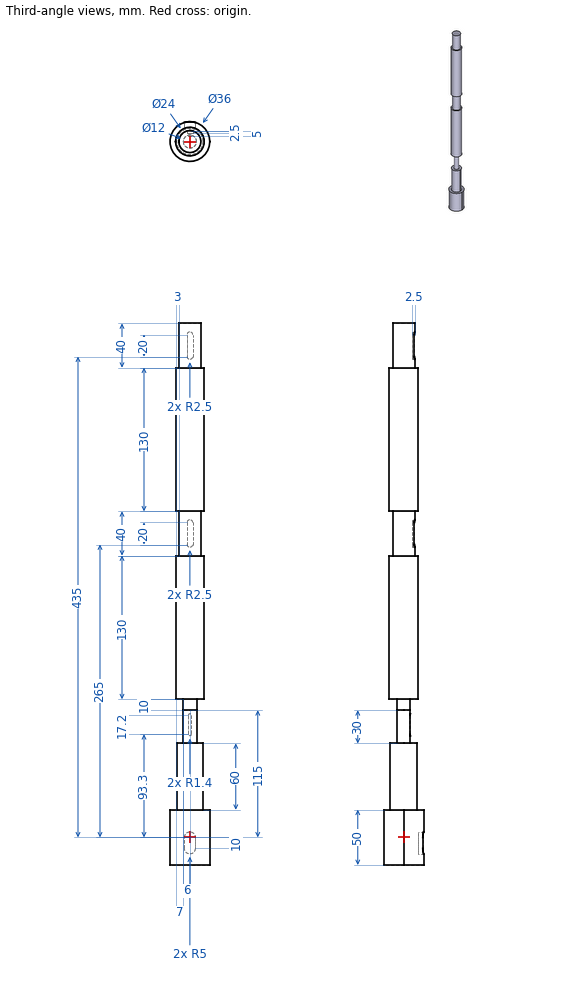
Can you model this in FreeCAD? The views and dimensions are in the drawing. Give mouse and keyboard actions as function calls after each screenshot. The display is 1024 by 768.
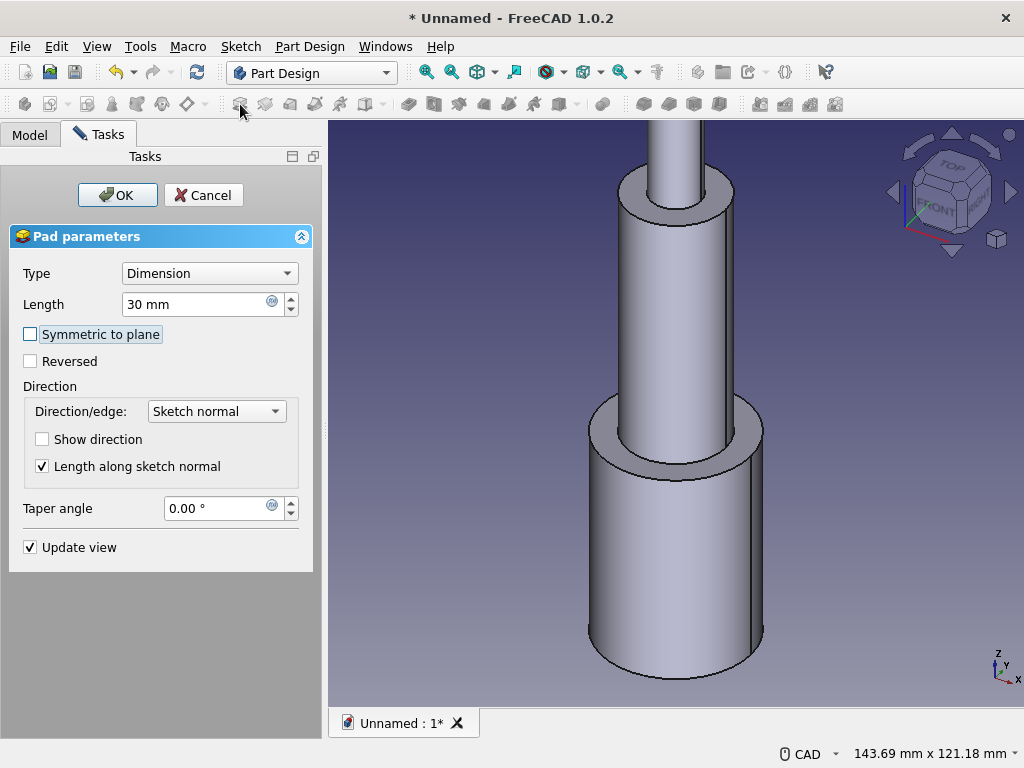
click(118, 195)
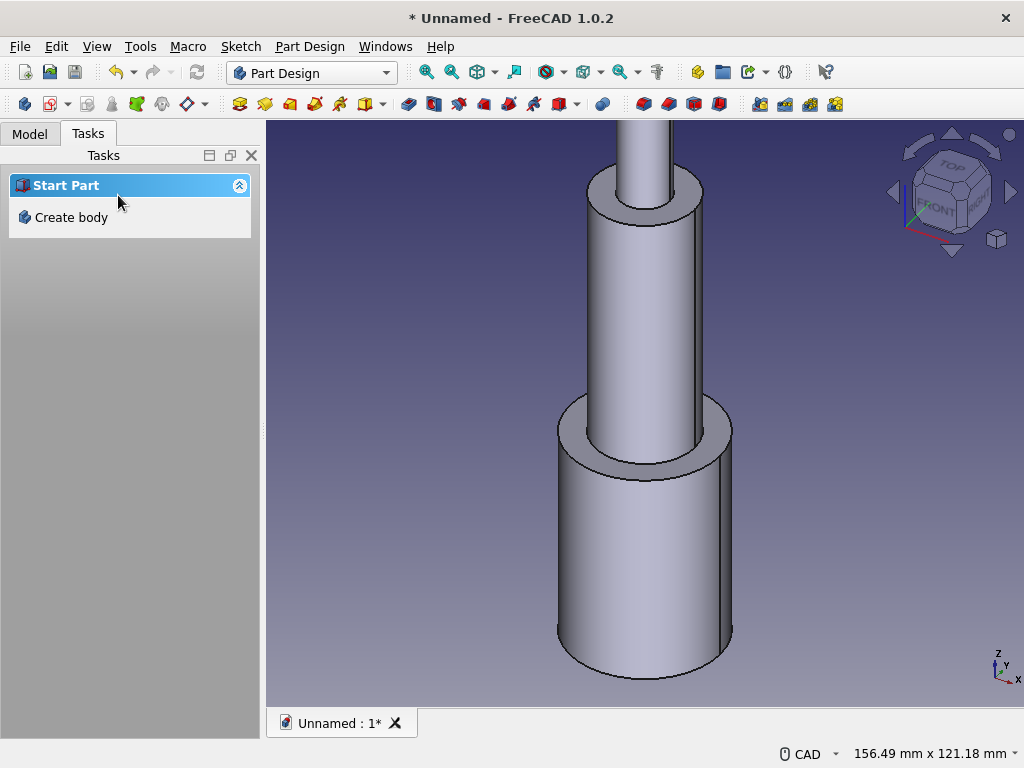
click(427, 72)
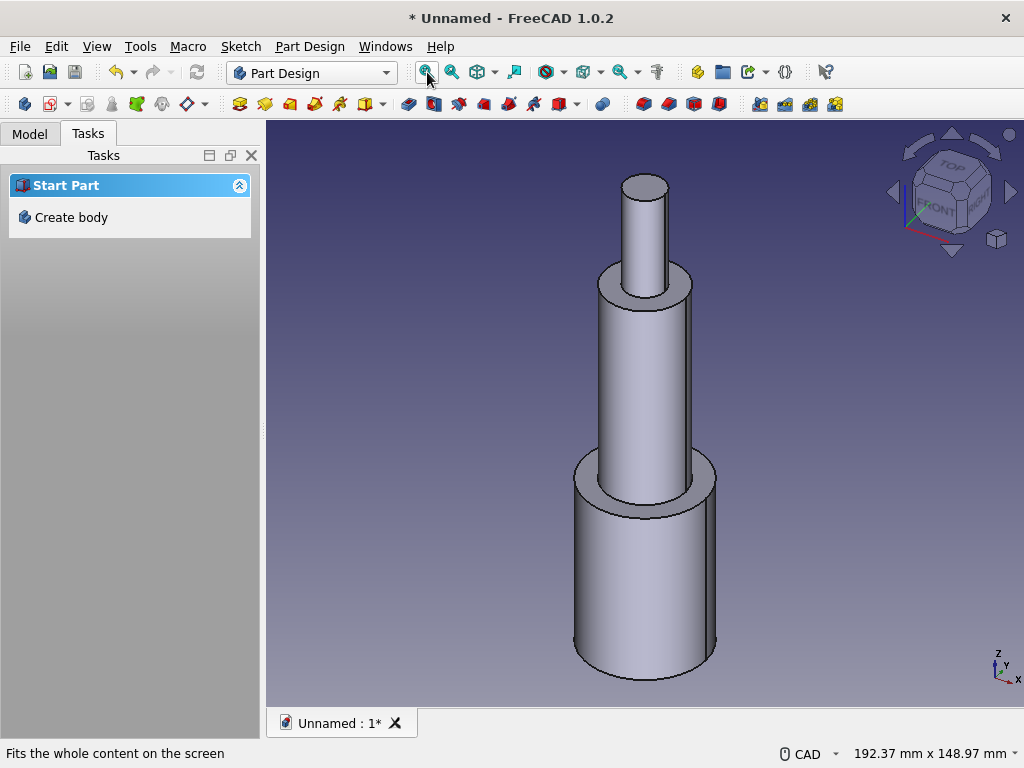
click(30, 134)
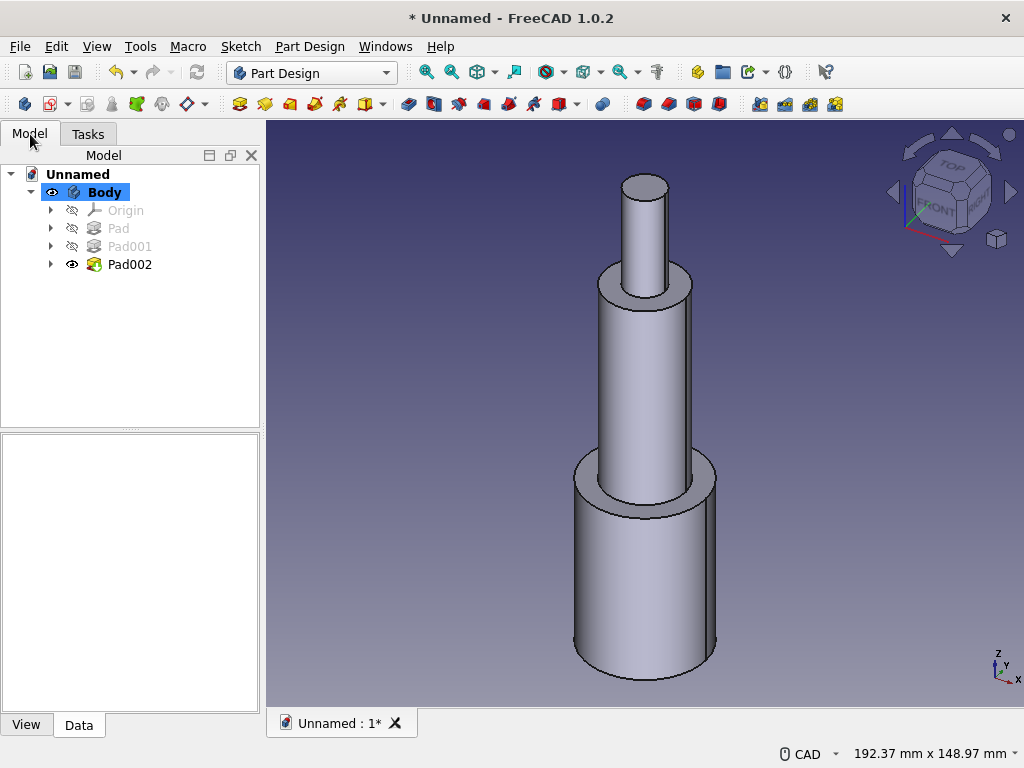
click(51, 210)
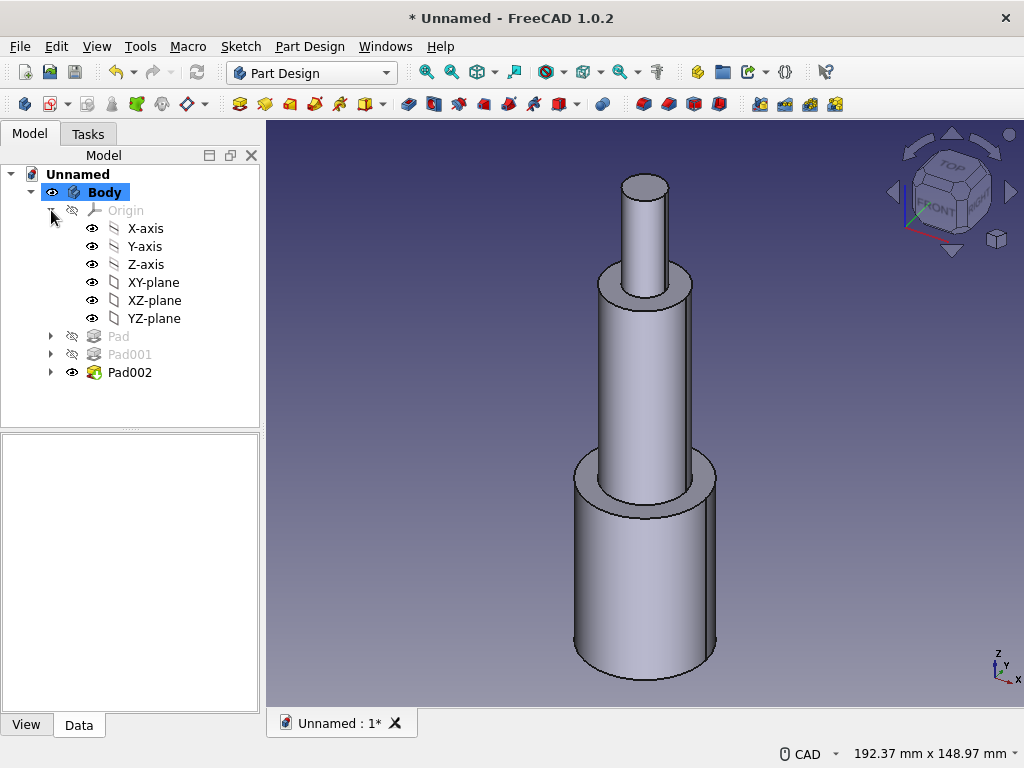
click(137, 300)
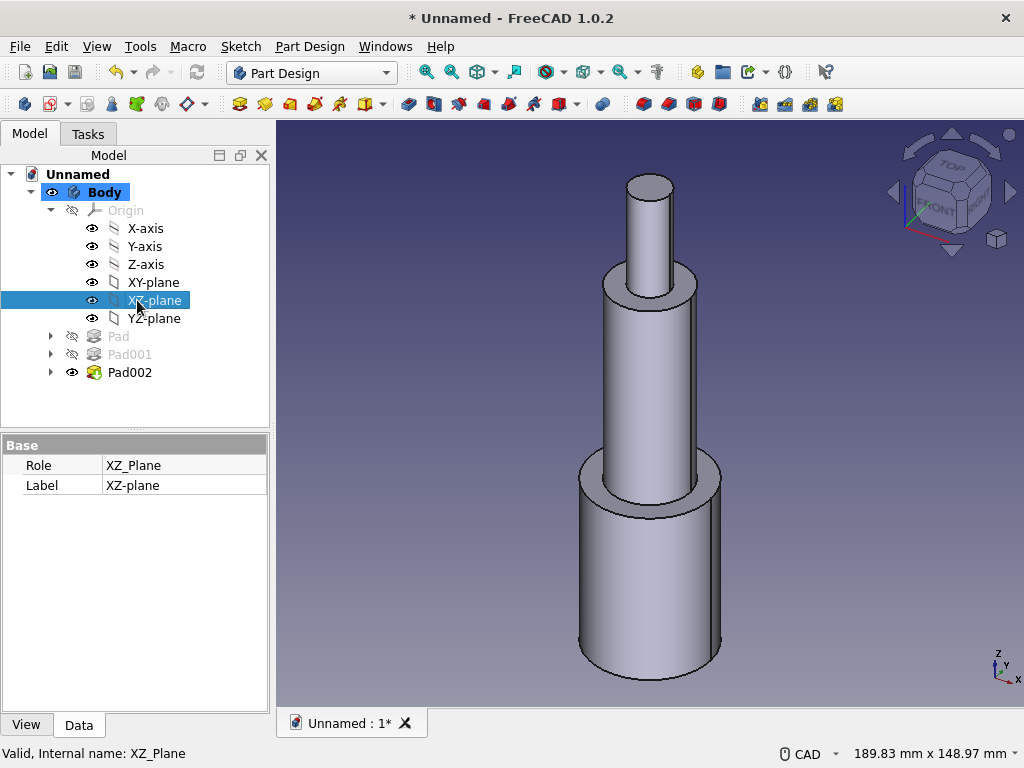
click(186, 104)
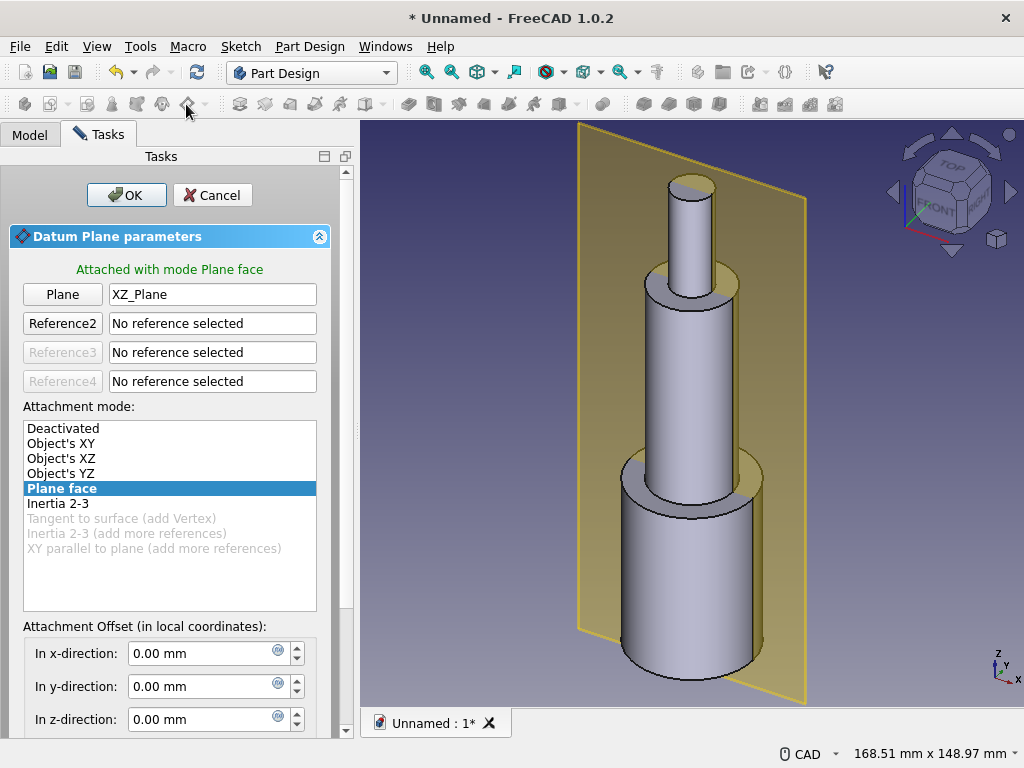
triple_click(210, 720)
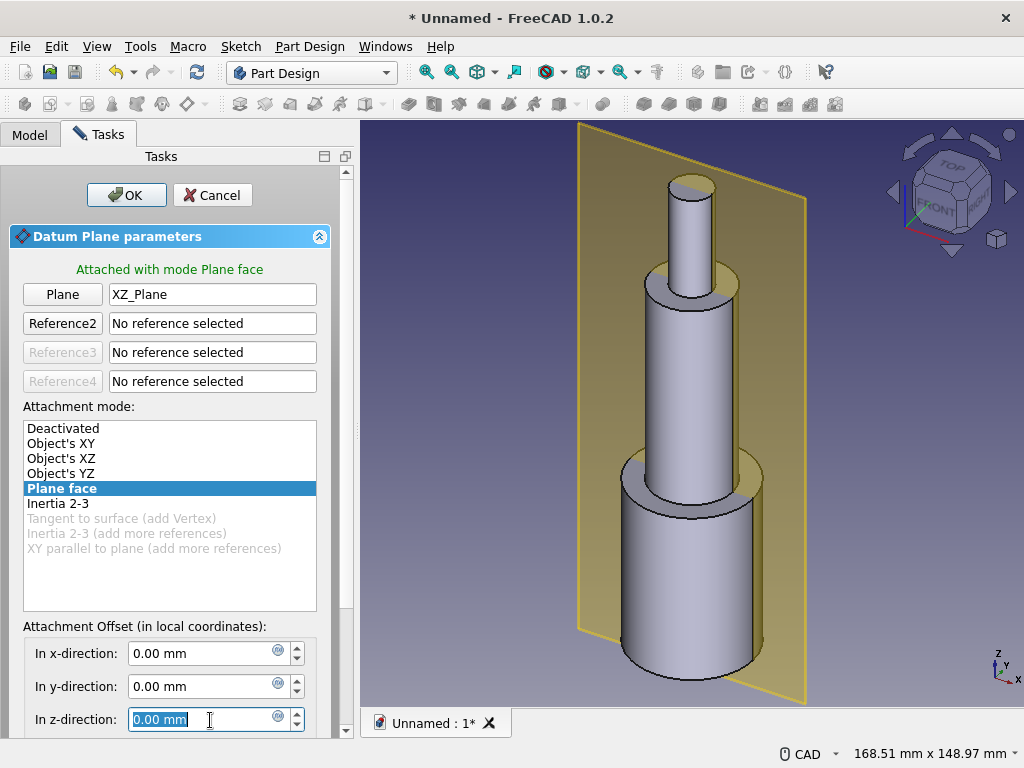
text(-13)
key(Tab)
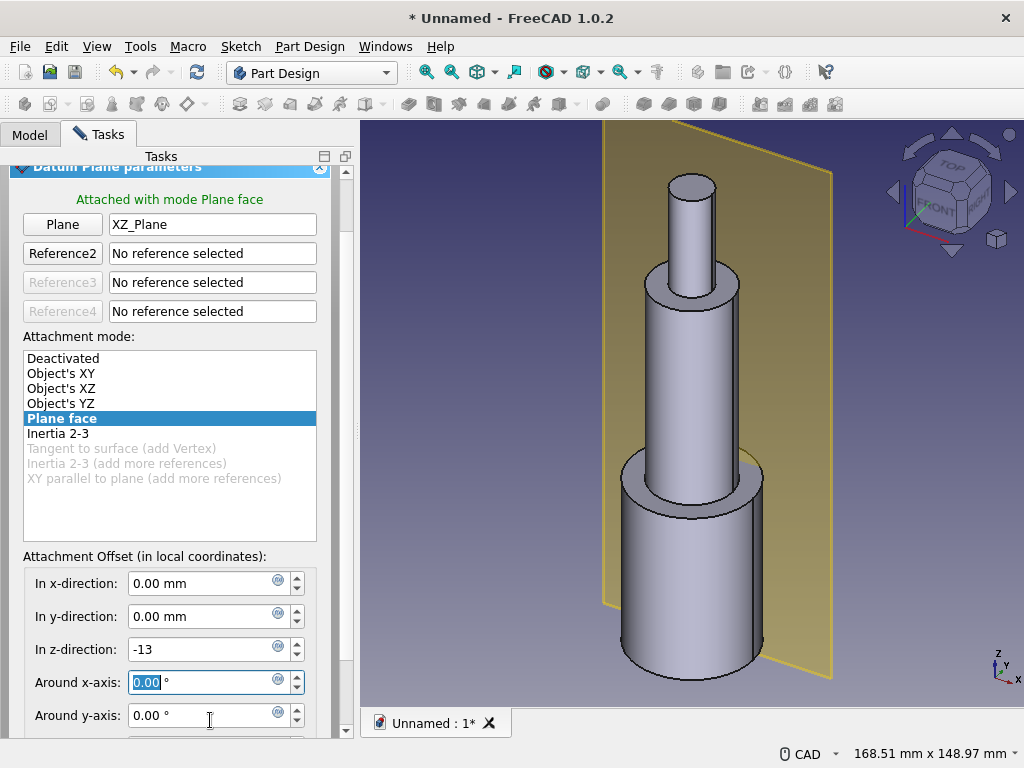
scroll(346, 452, up, 2)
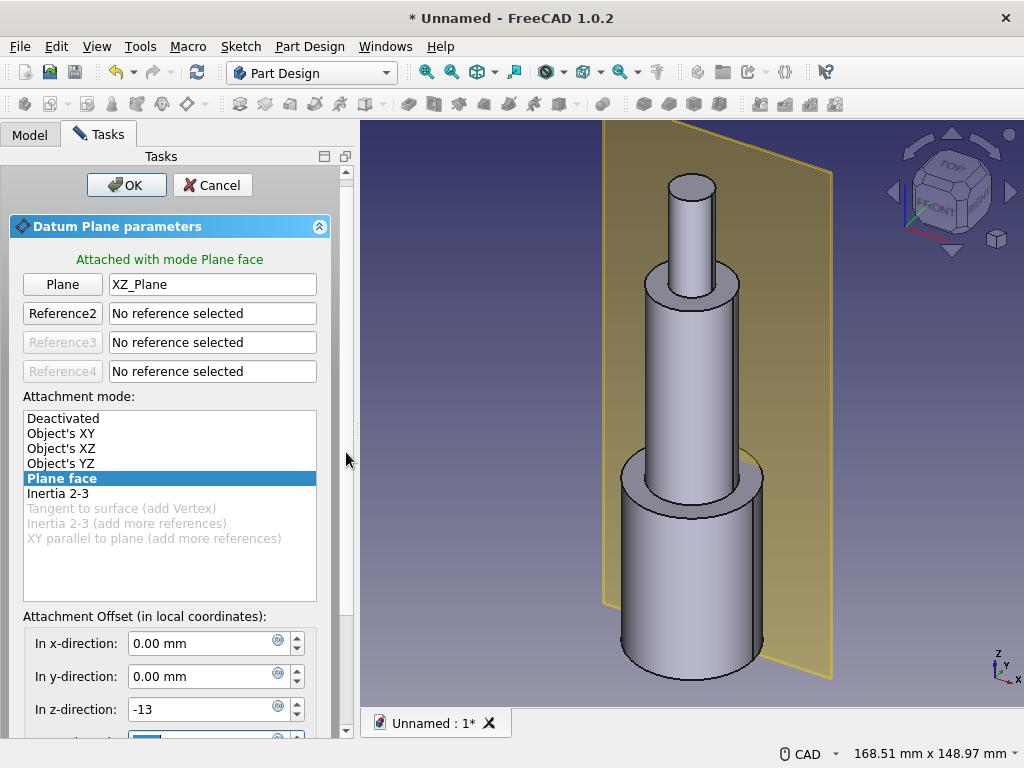
click(127, 195)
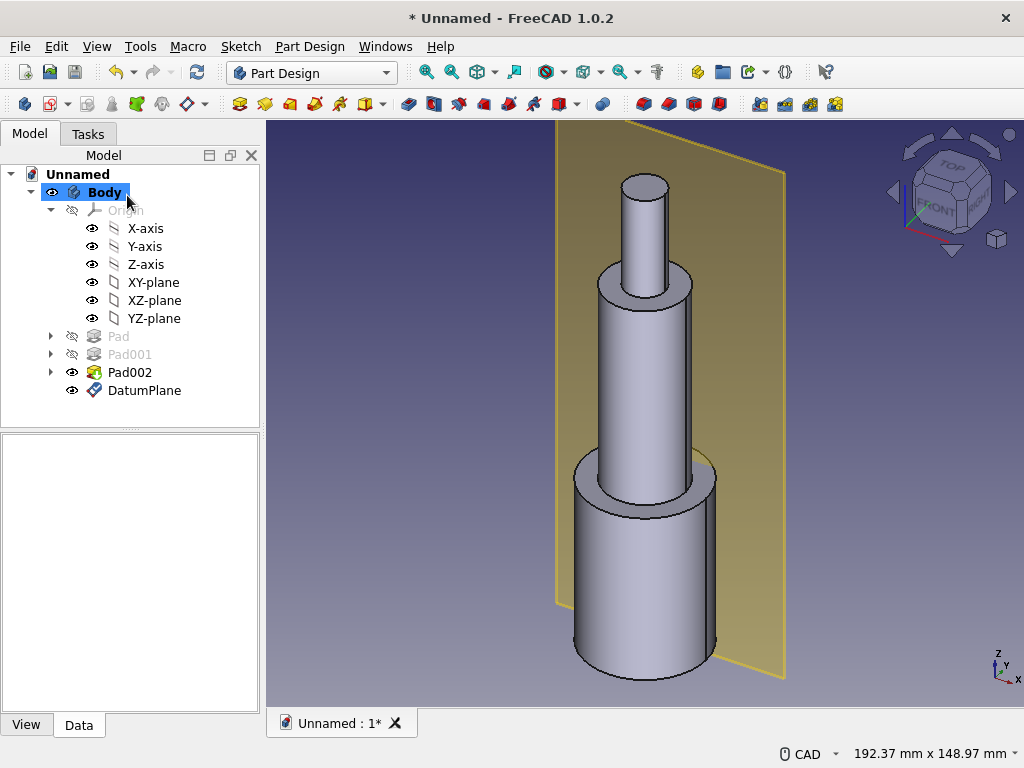
click(117, 390)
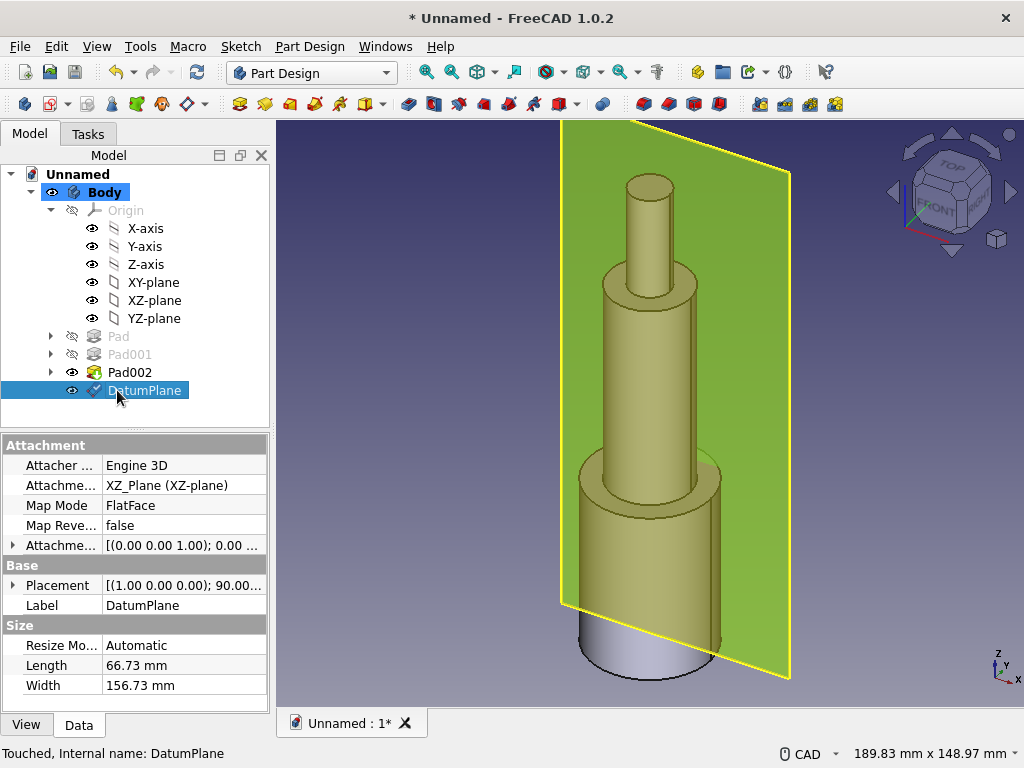
click(50, 104)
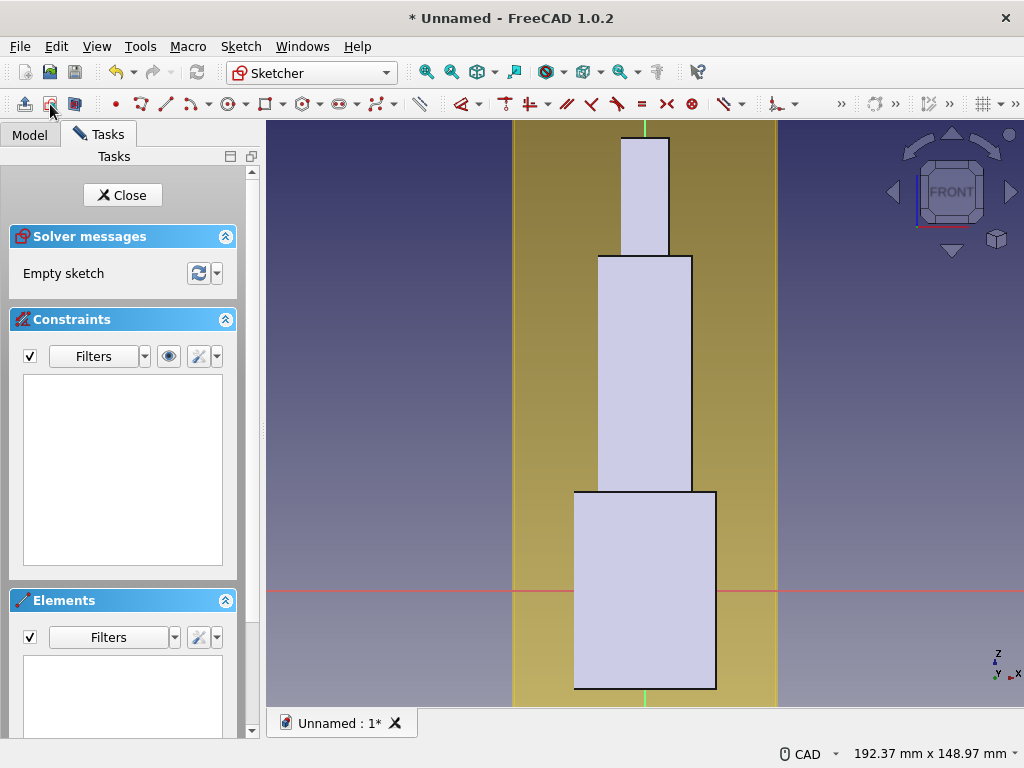
click(75, 104)